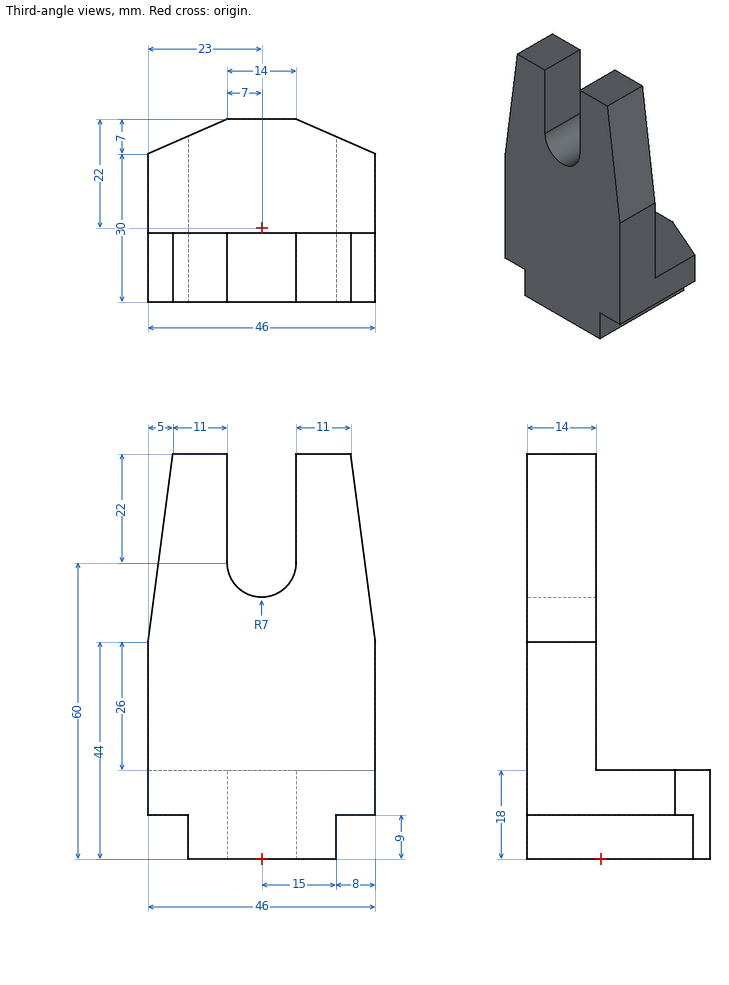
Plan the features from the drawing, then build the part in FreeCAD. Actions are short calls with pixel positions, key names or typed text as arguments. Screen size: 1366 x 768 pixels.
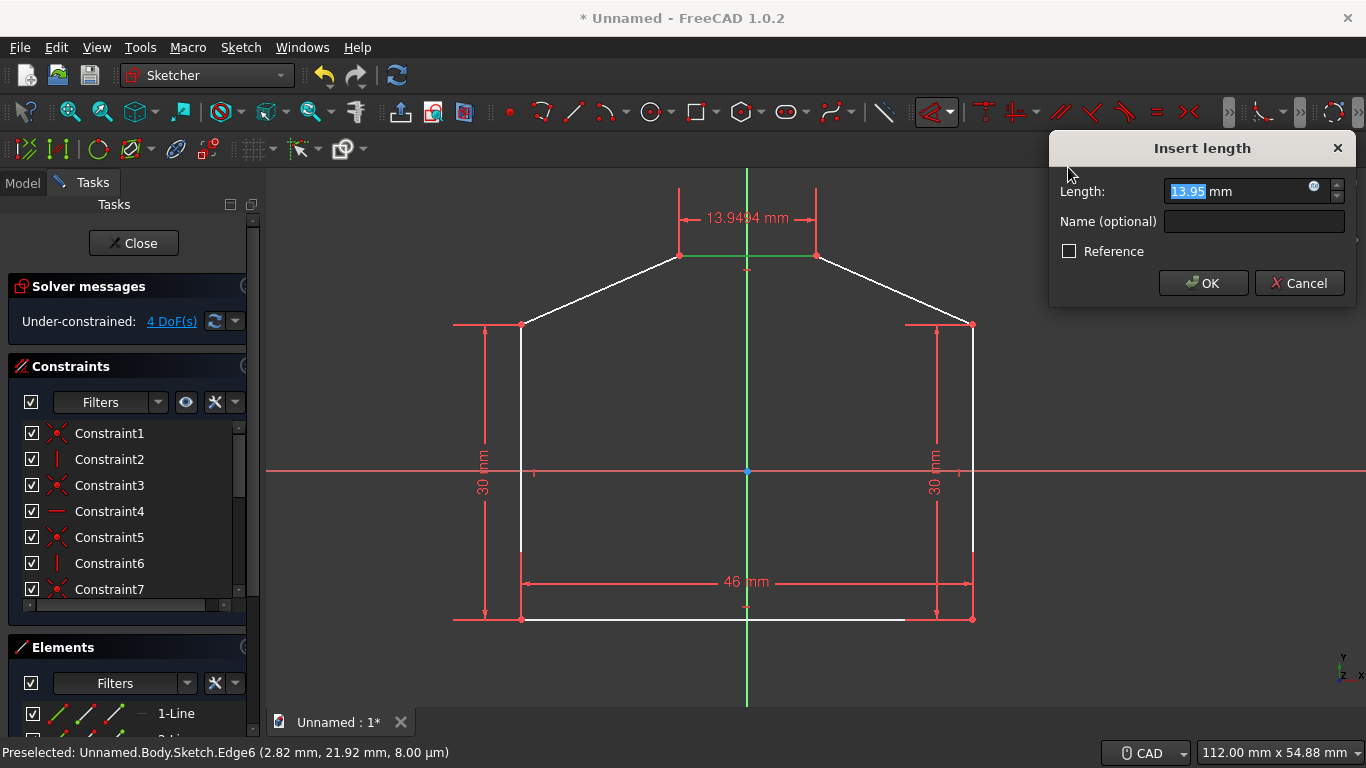
text(14)
key(Return)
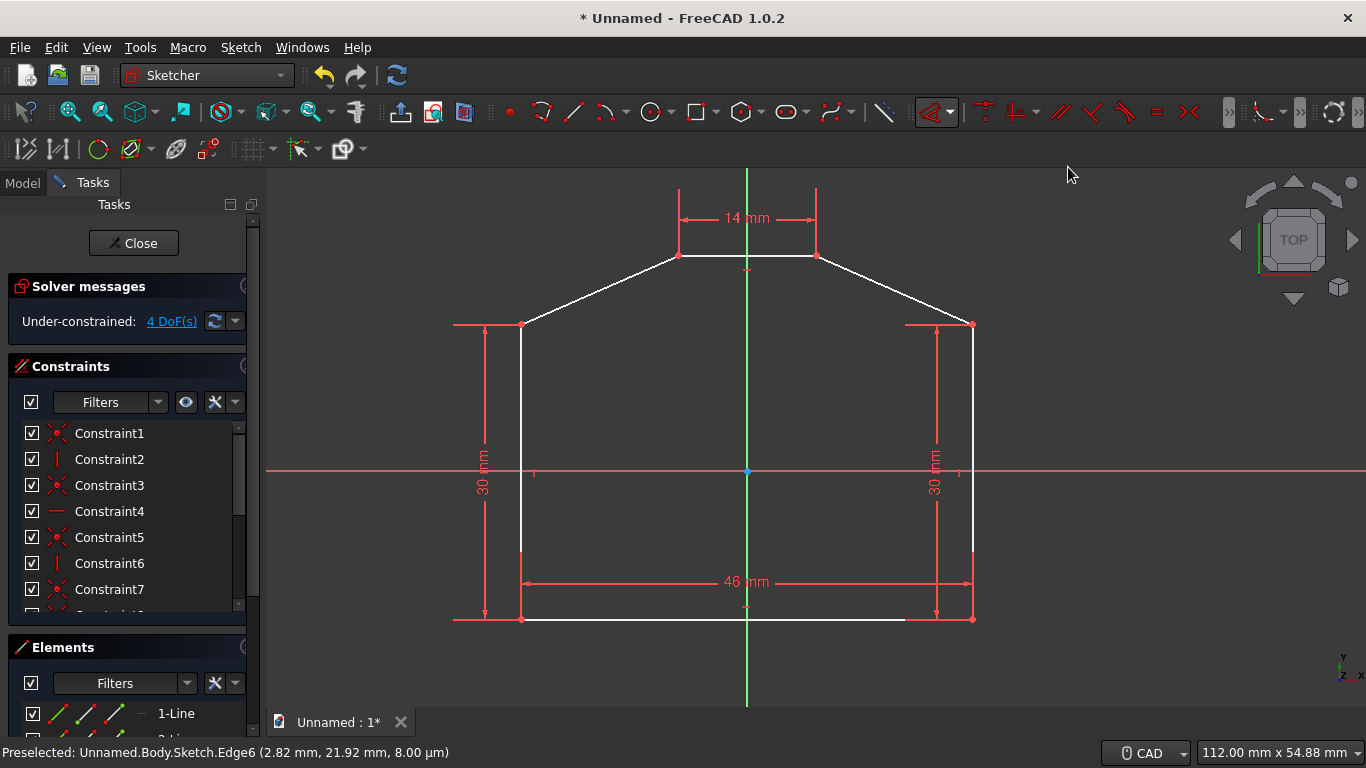
click(679, 256)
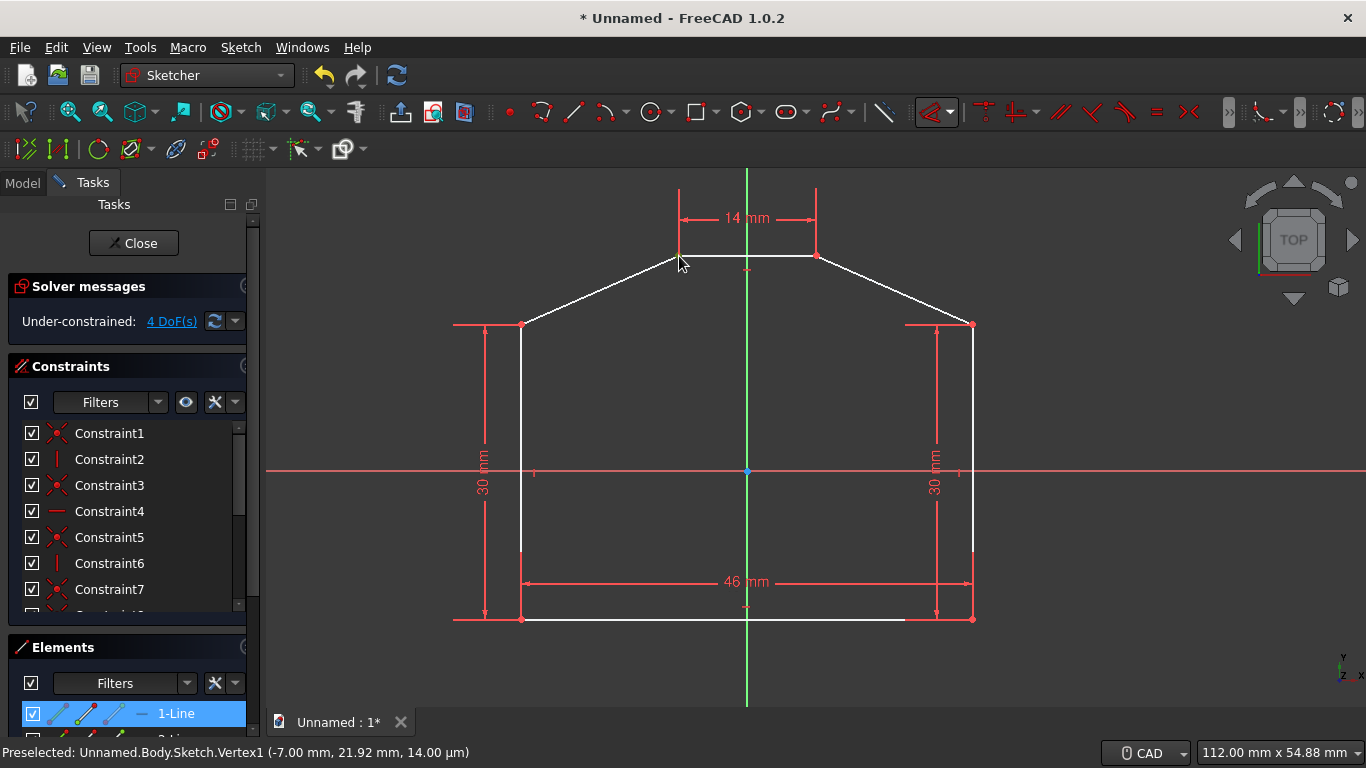
click(952, 112)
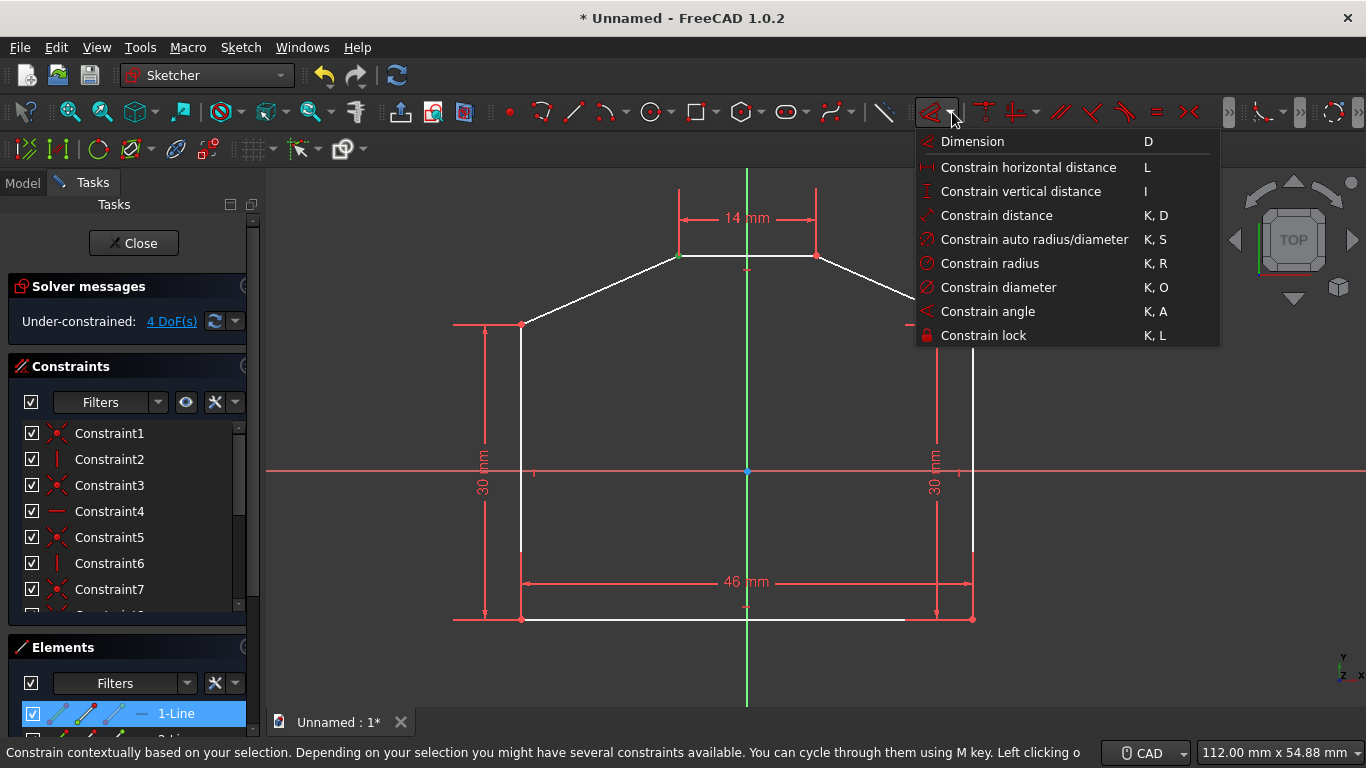
click(1068, 167)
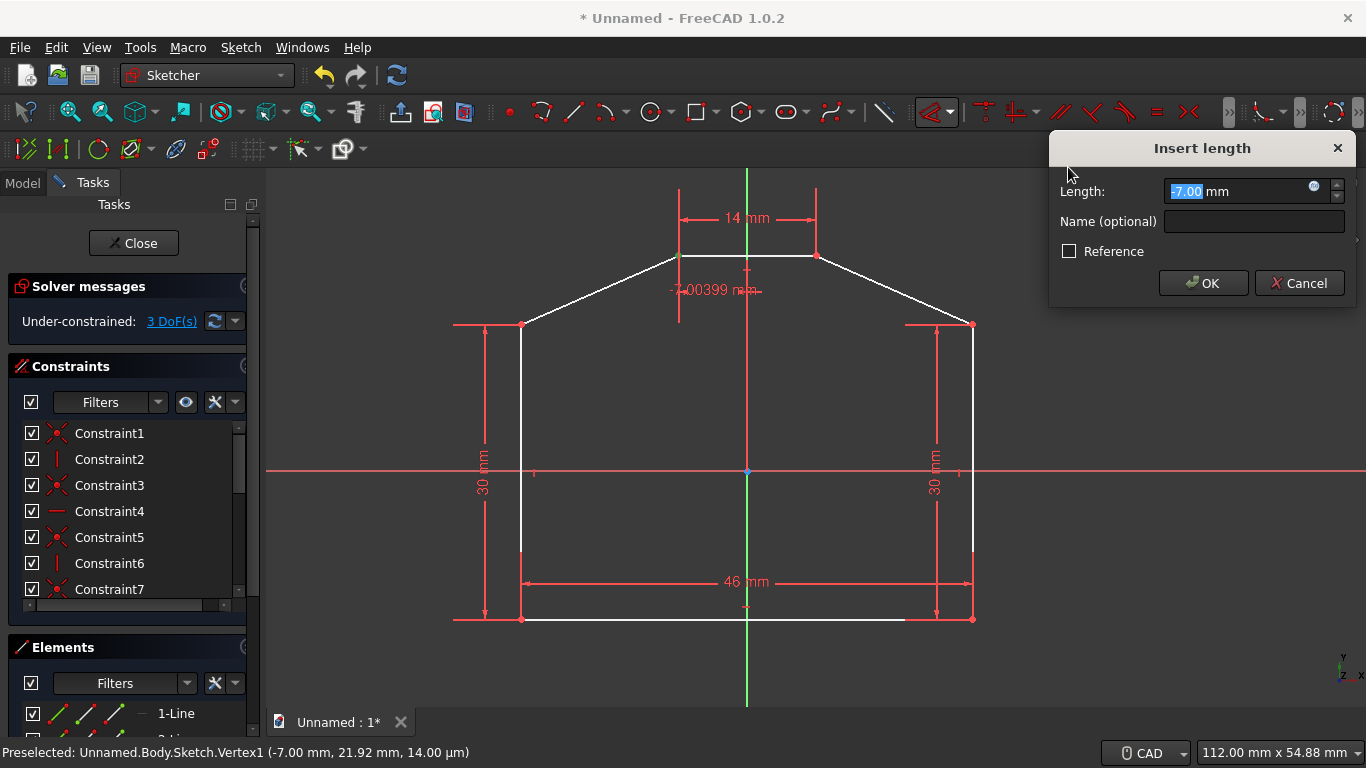
text(-7)
key(Return)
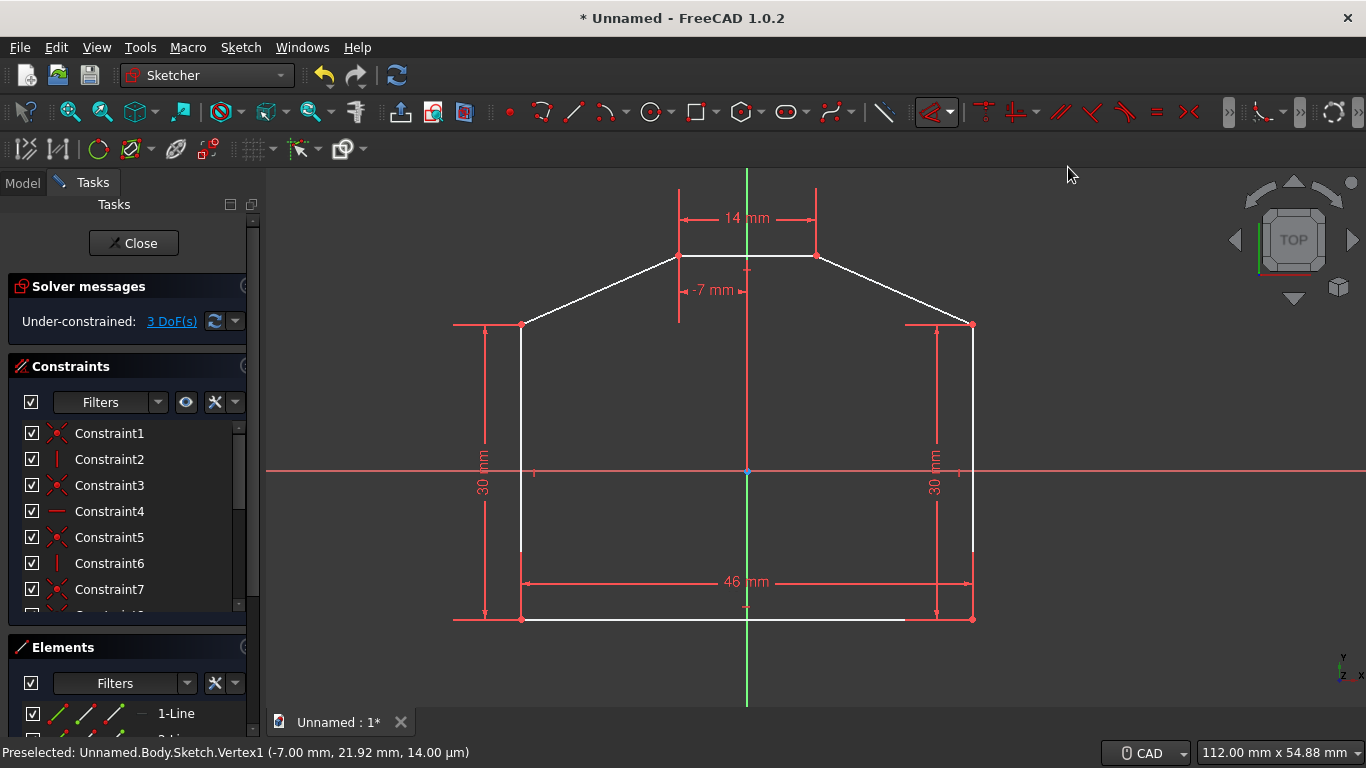
click(631, 277)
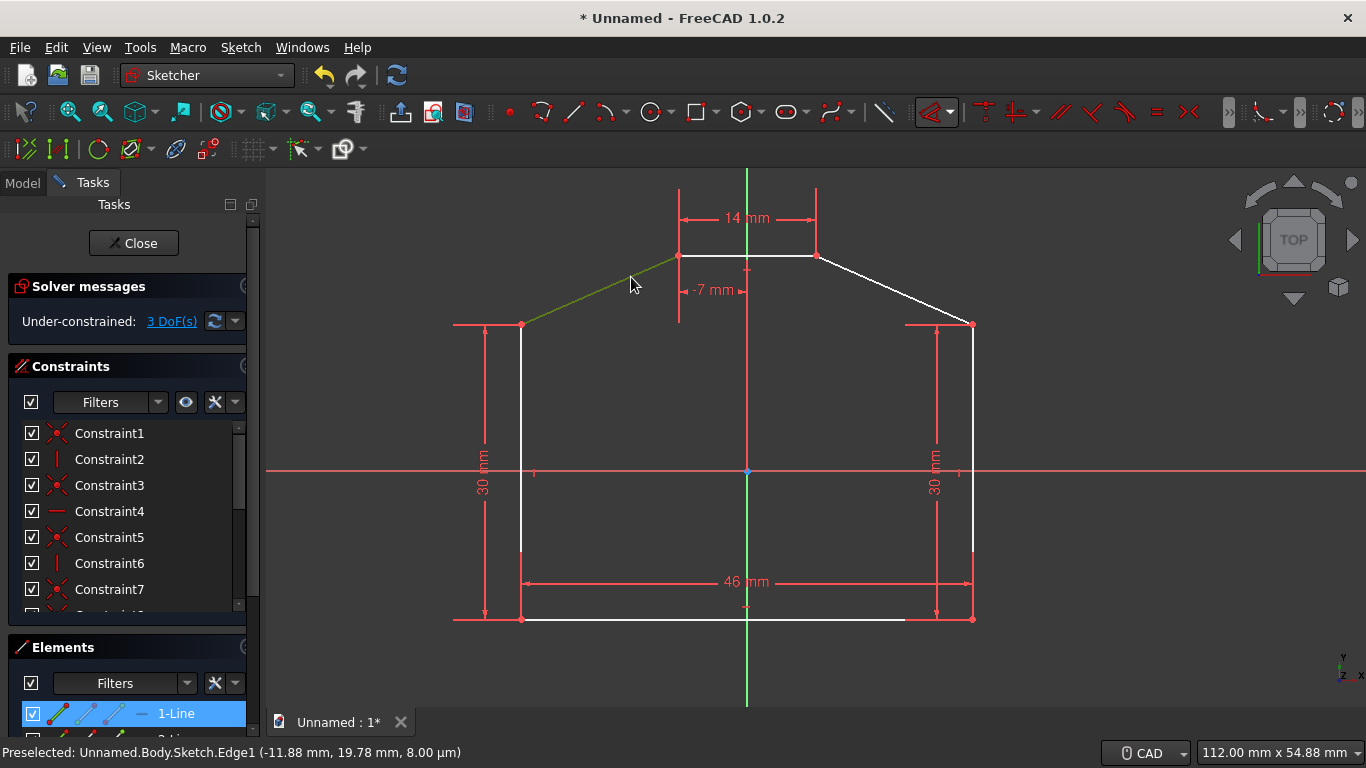
click(952, 112)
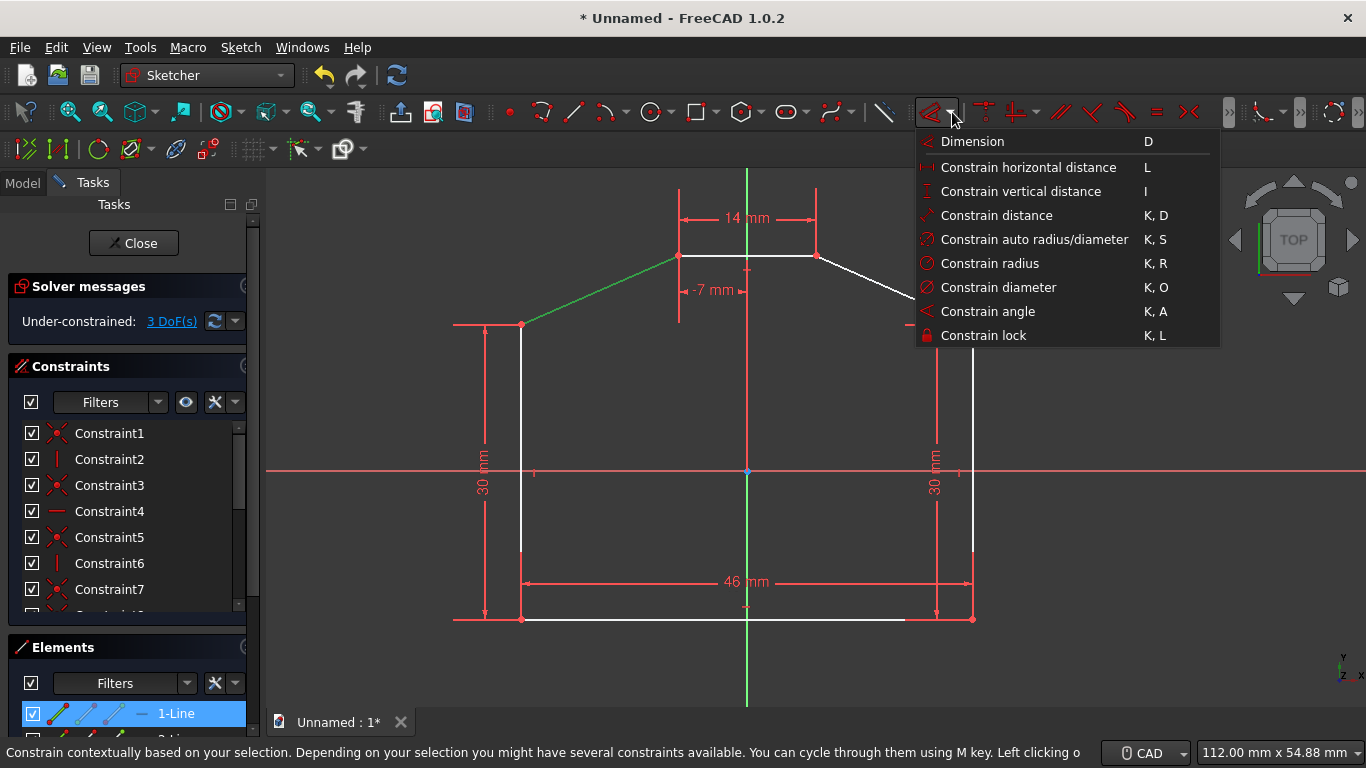
click(1068, 191)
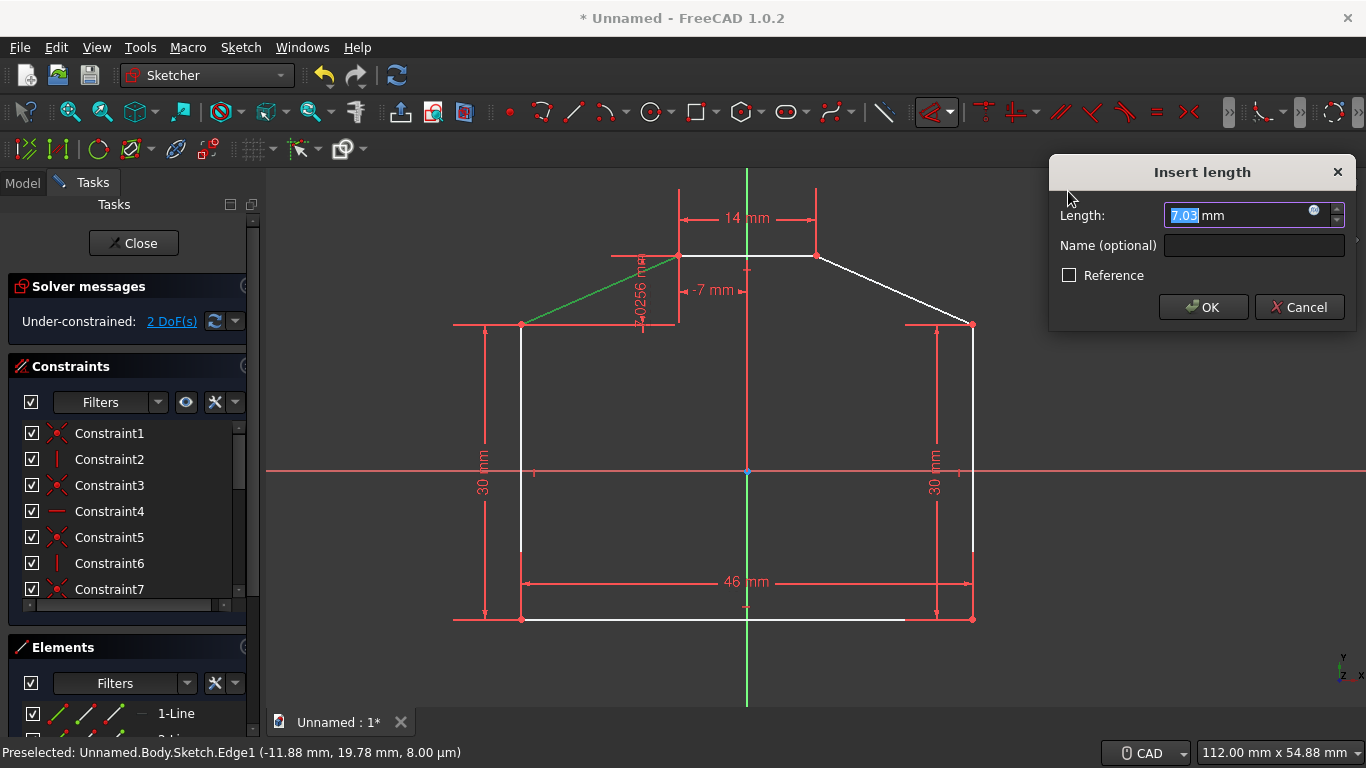
text(7)
key(Return)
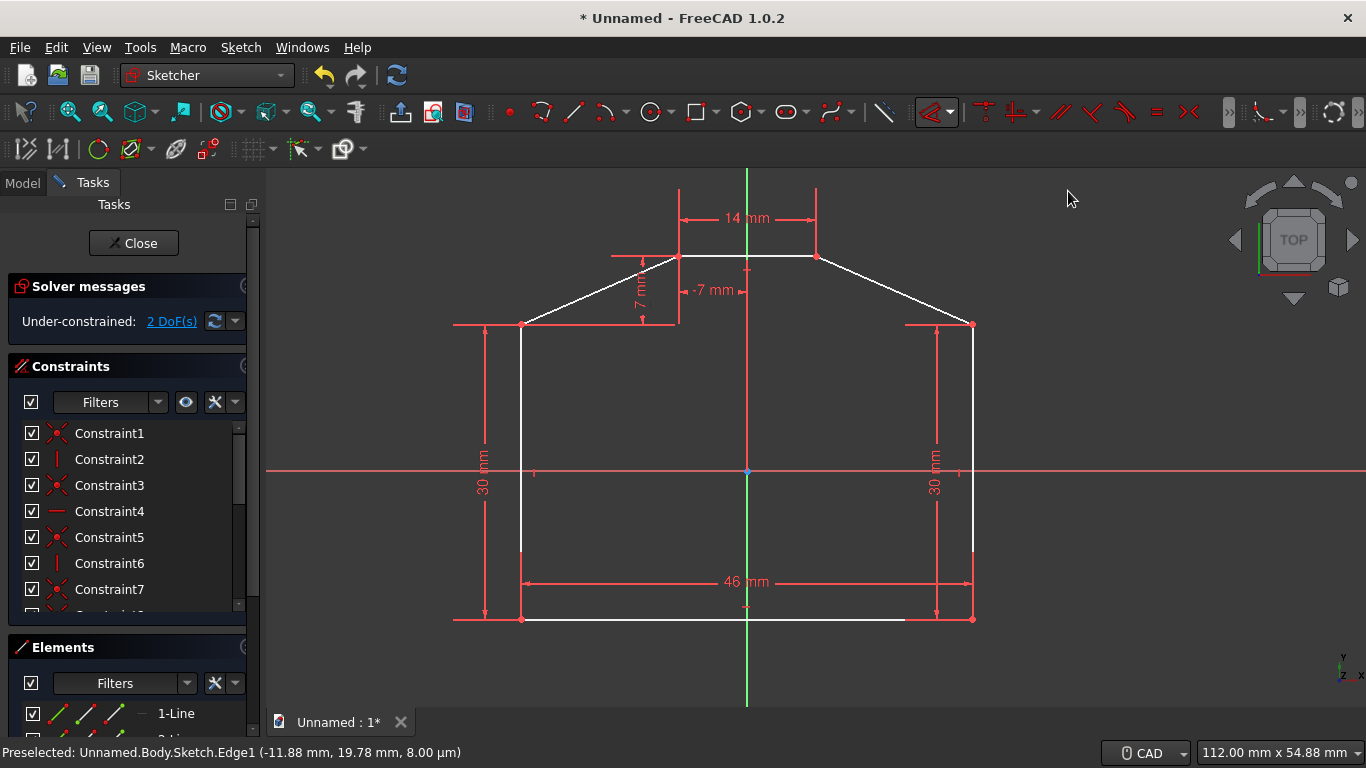
click(679, 256)